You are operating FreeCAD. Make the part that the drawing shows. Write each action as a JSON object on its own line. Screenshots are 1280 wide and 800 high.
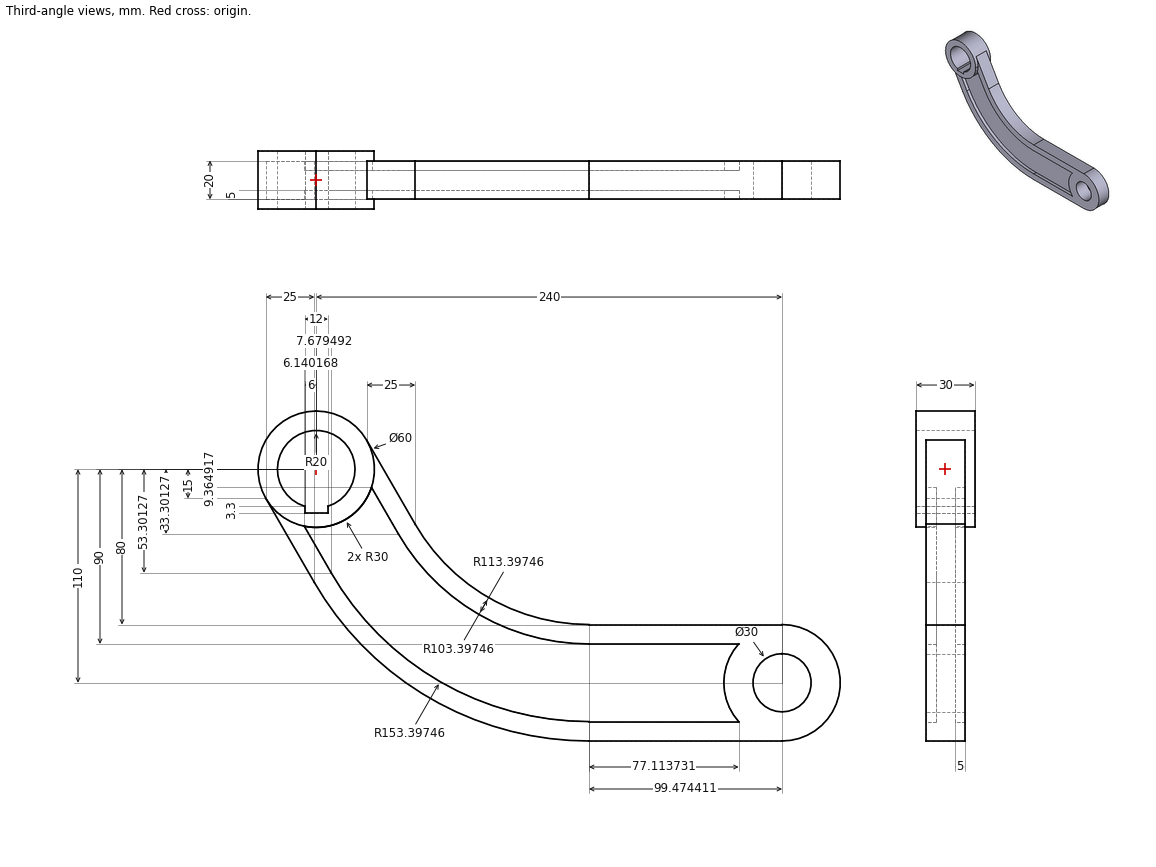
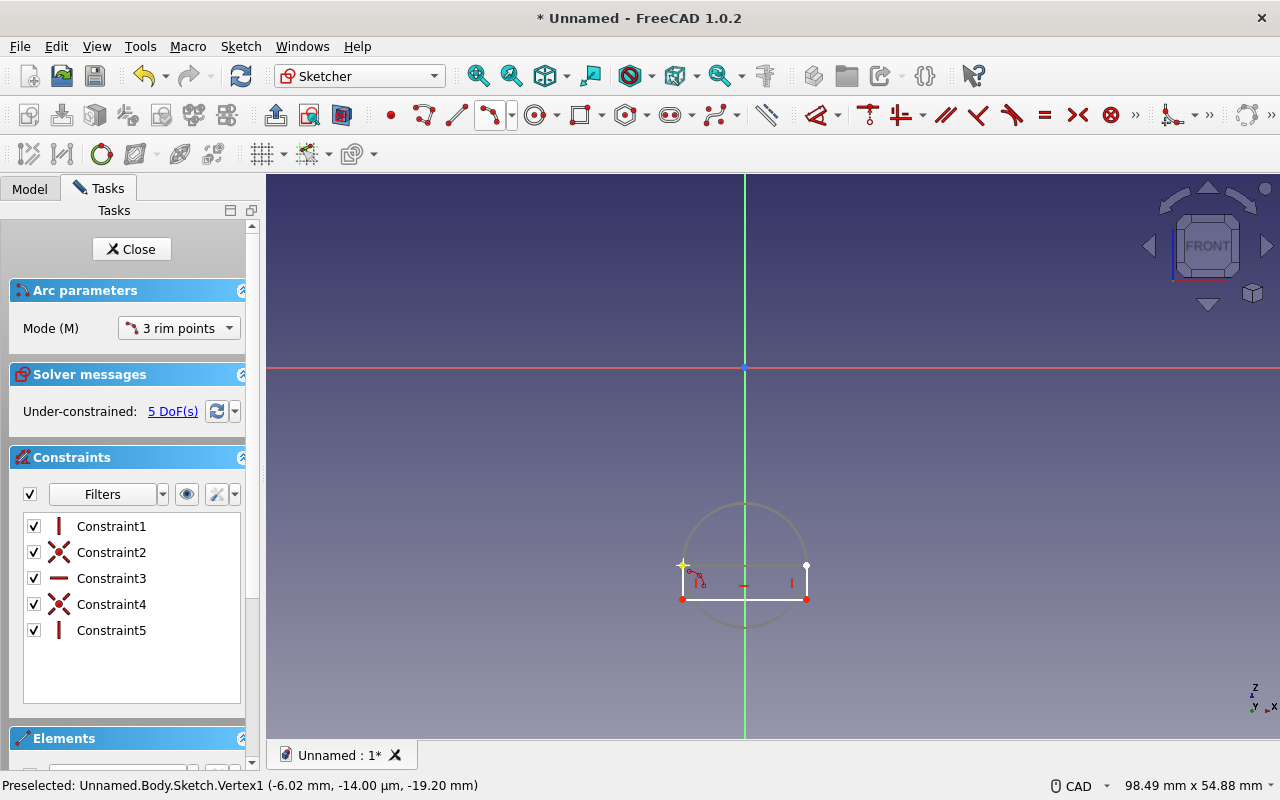
{"action": "scroll", "coordinate": [656, 565], "scroll_direction": "down", "scroll_amount": 3}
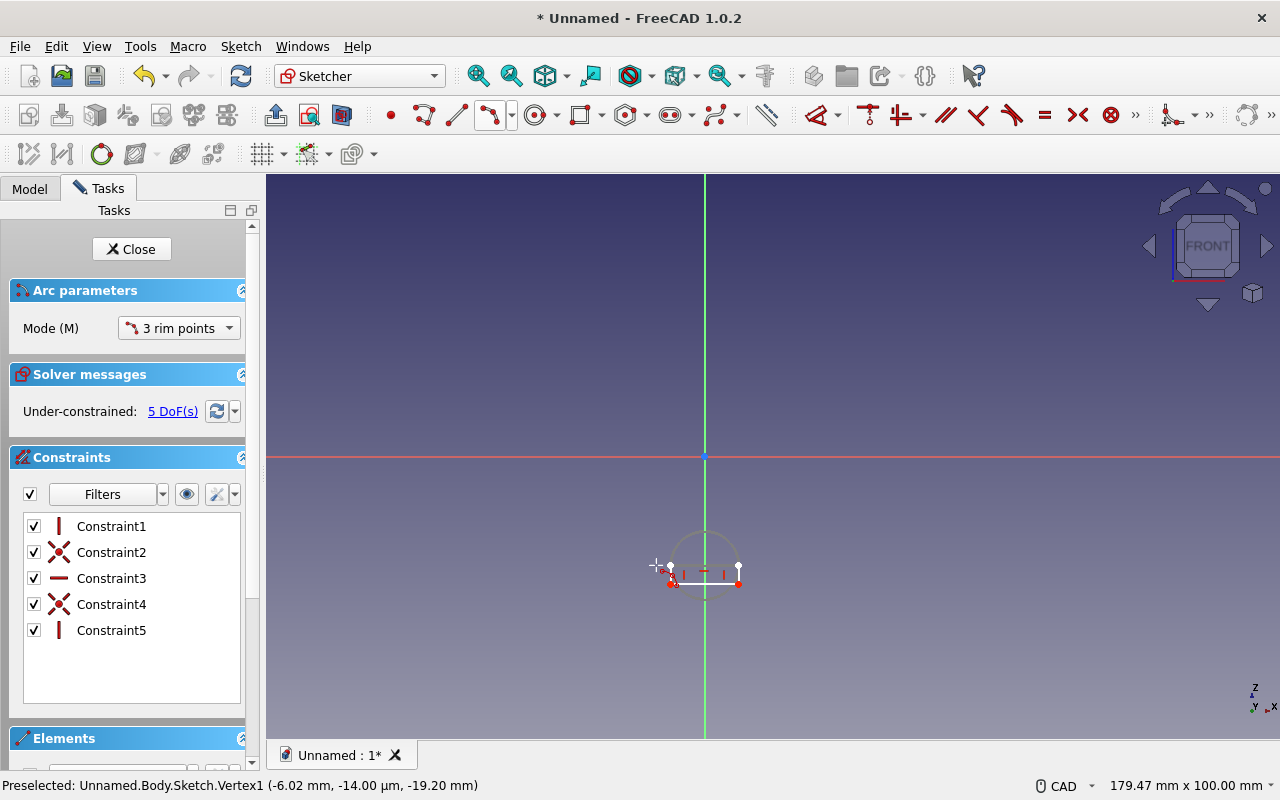
{"action": "left_click", "coordinate": [766, 362]}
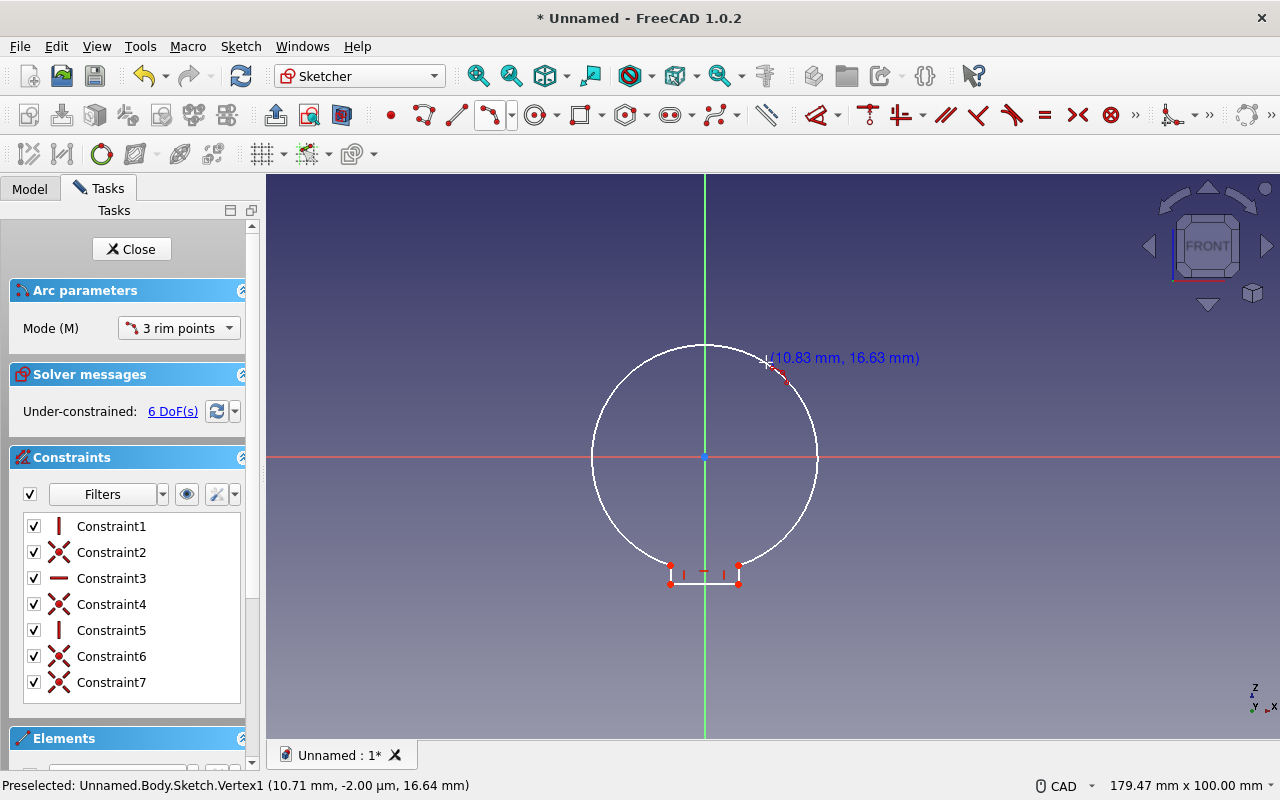
{"action": "left_click", "coordinate": [534, 116]}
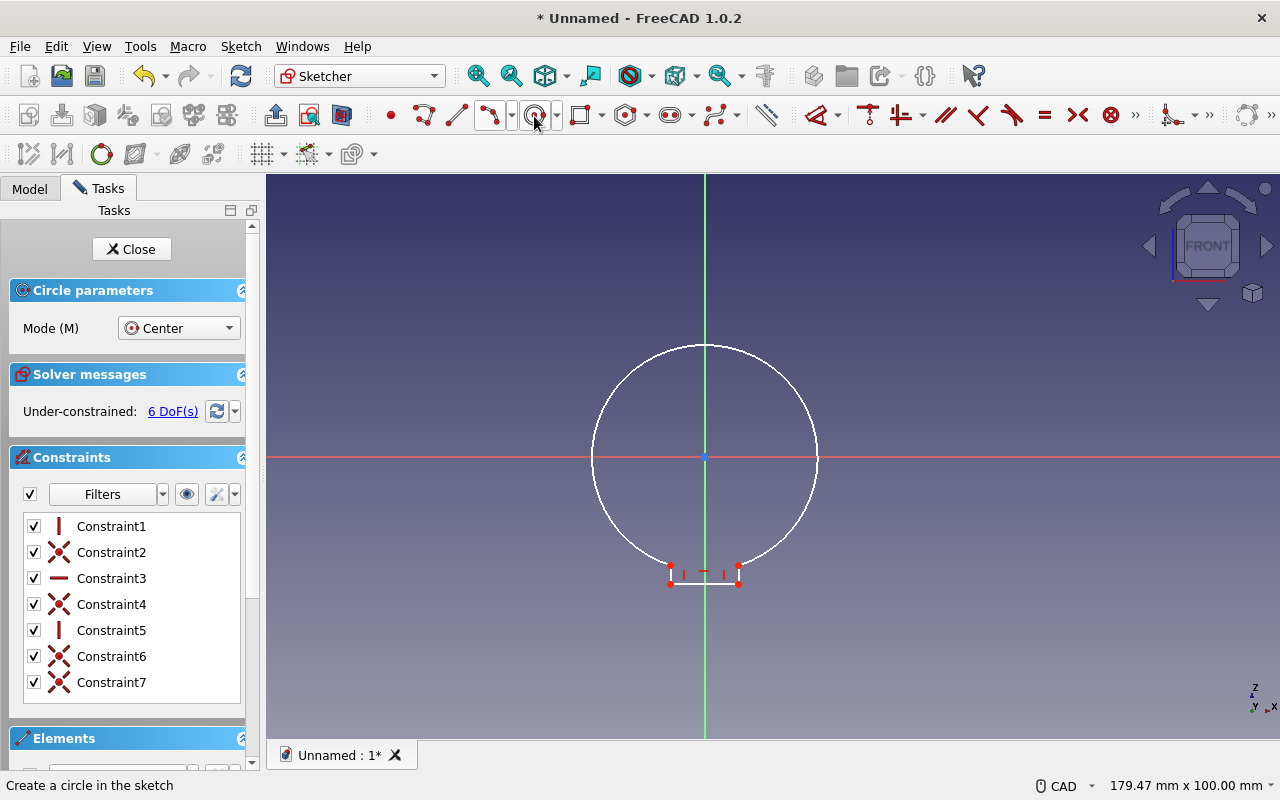
{"action": "left_click", "coordinate": [705, 457]}
{"action": "mouse_move", "coordinate": [825, 337]}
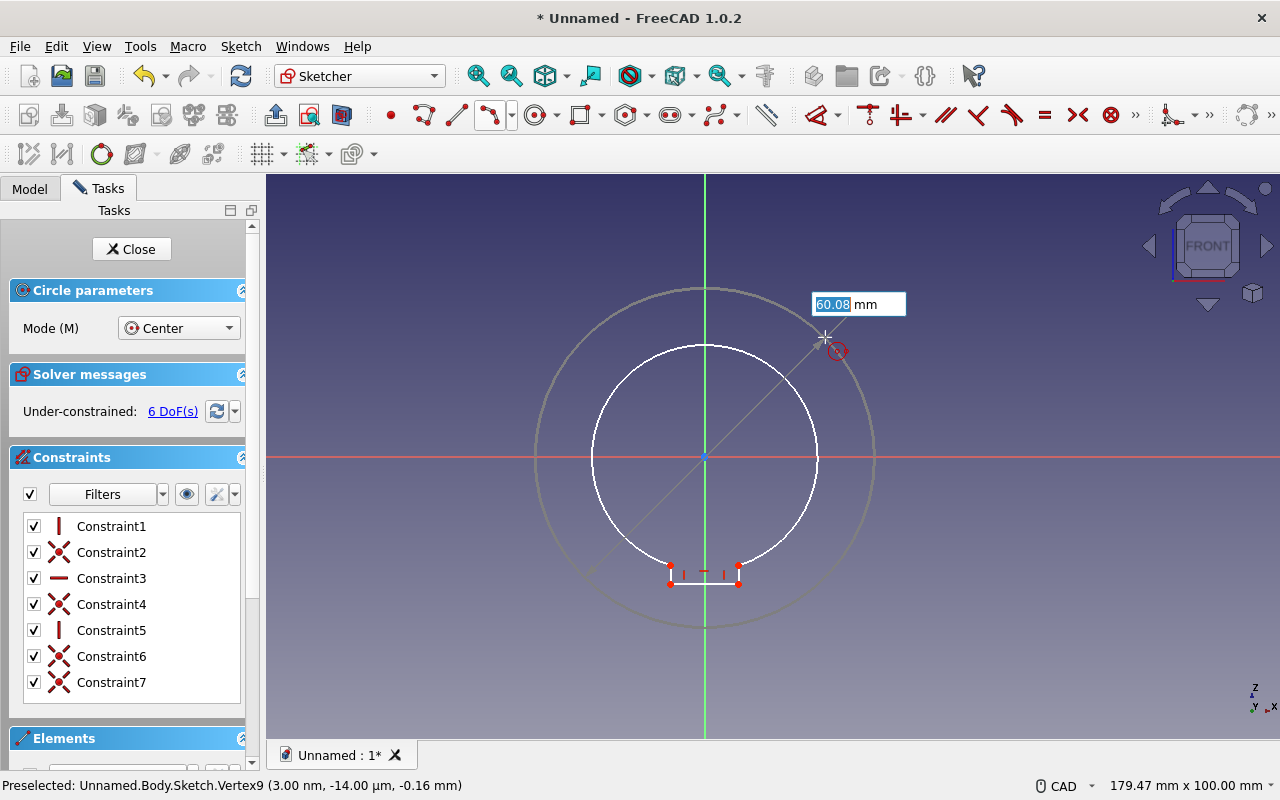
{"action": "type", "text": "60"}
{"action": "key", "text": "Return"}
{"action": "key", "text": "Escape"}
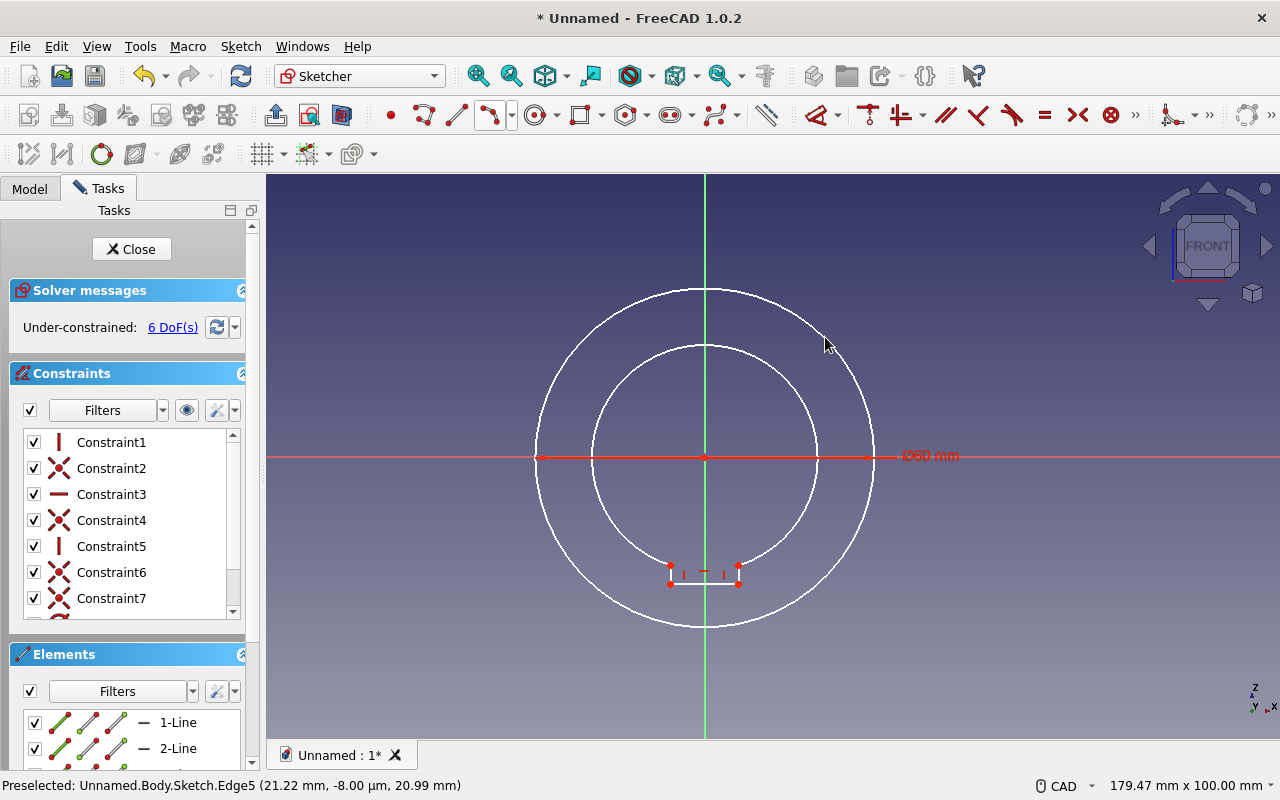
{"action": "left_click_drag", "start_coordinate": [695, 447], "coordinate": [715, 468]}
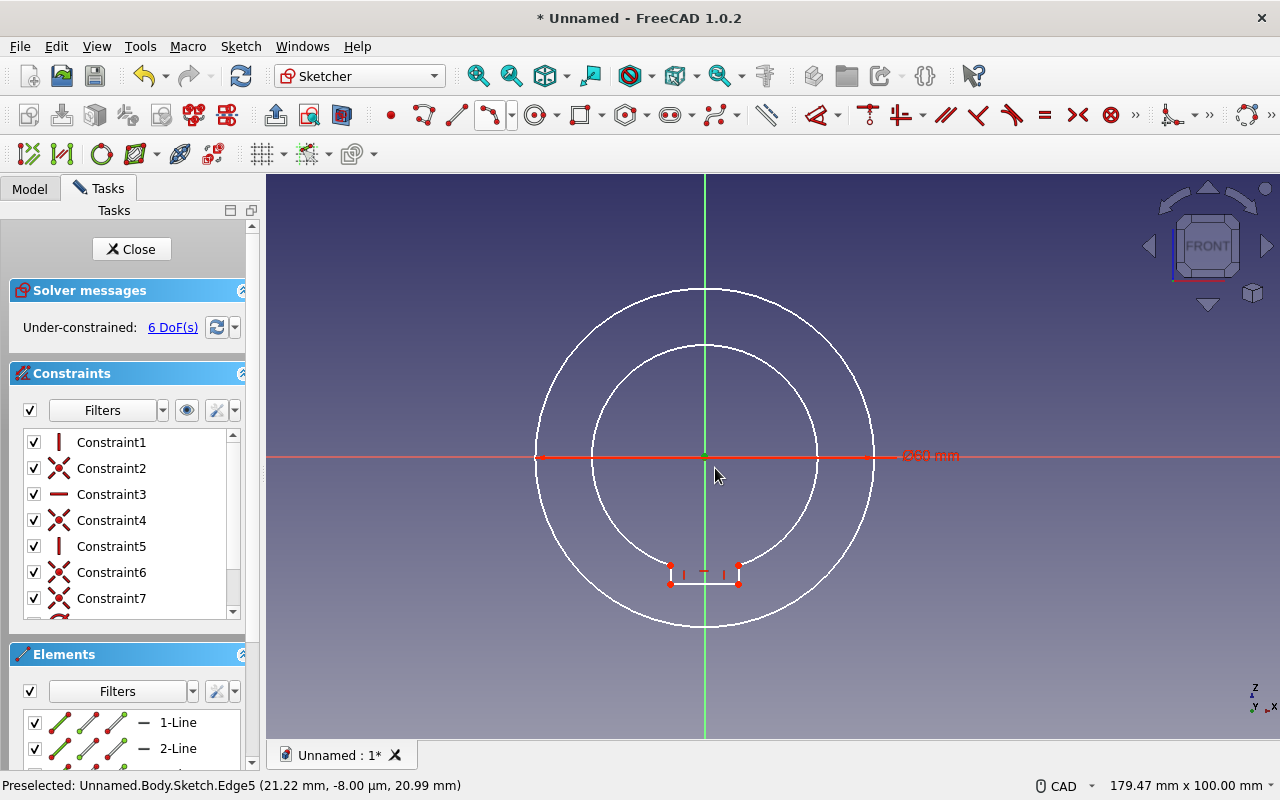
{"action": "left_click", "coordinate": [868, 116]}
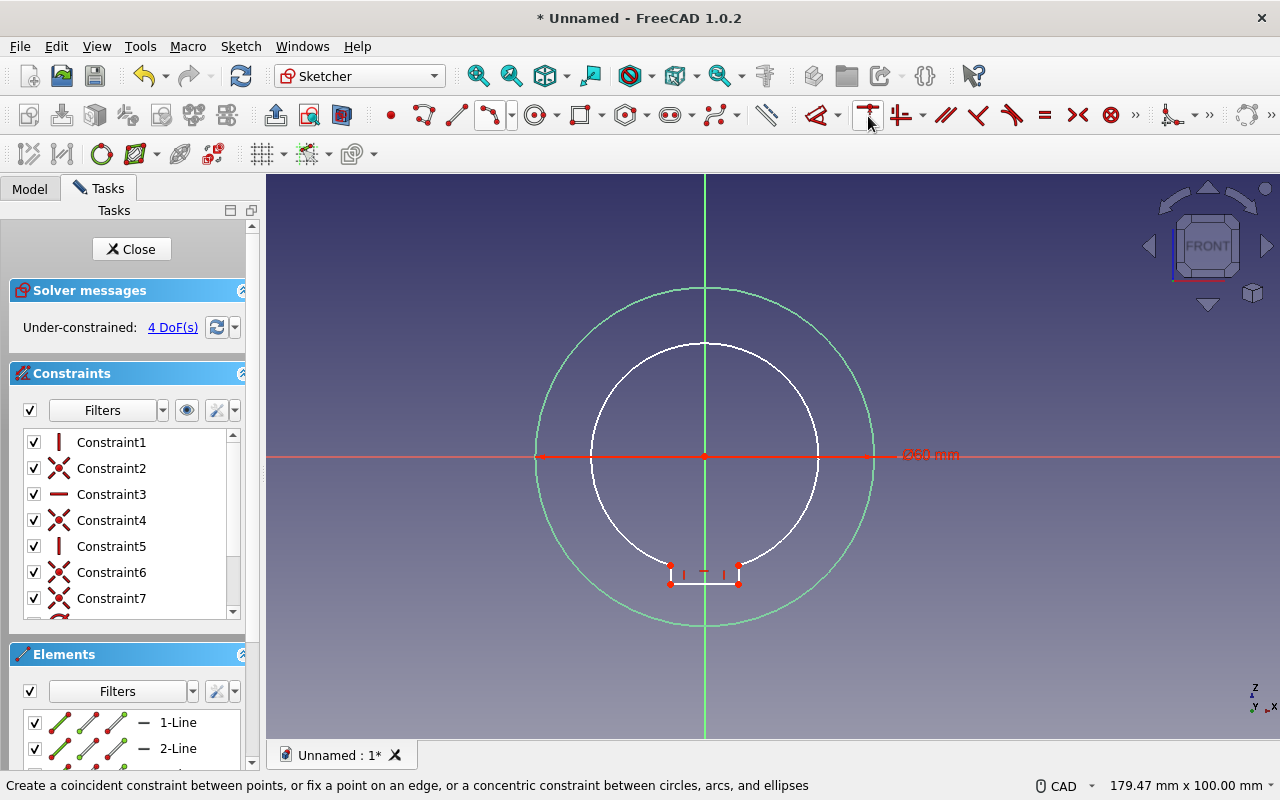
{"action": "left_click", "coordinate": [816, 116]}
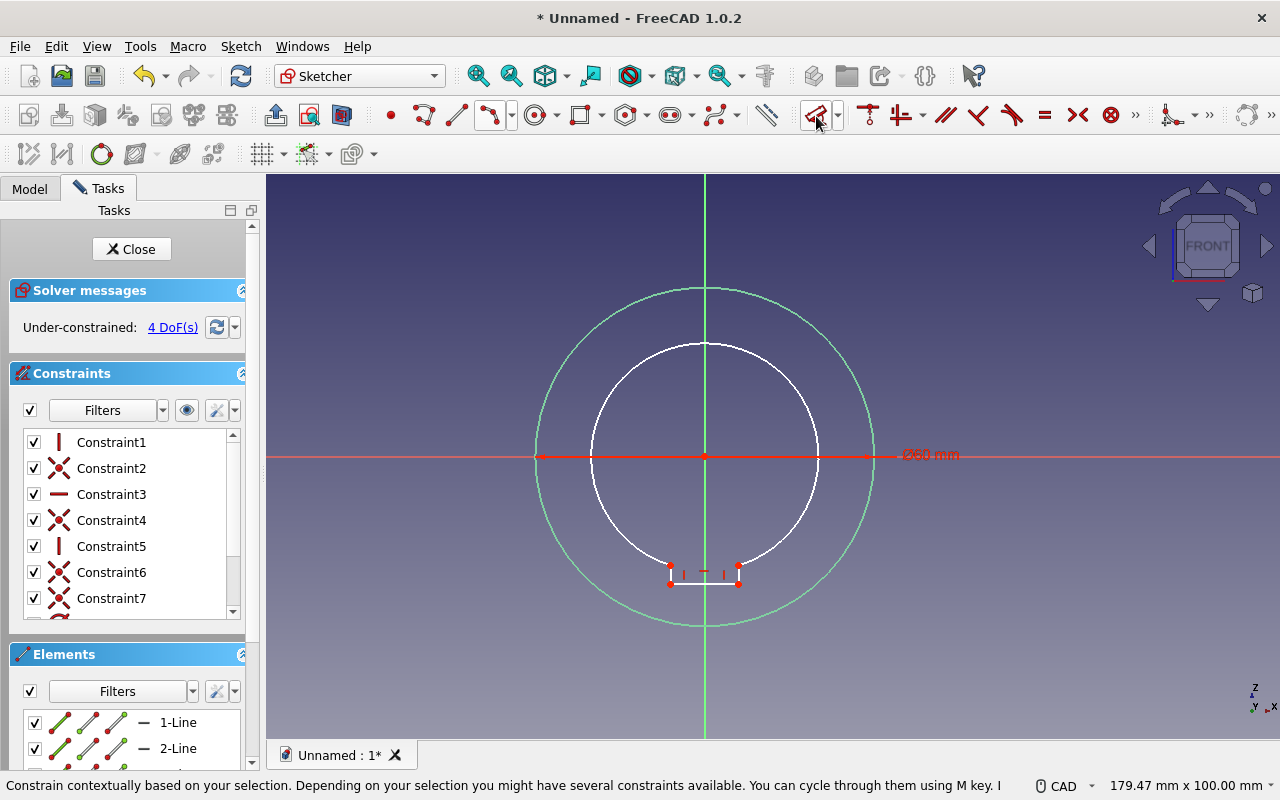
{"action": "left_click", "coordinate": [808, 409]}
{"action": "left_click", "coordinate": [837, 396]}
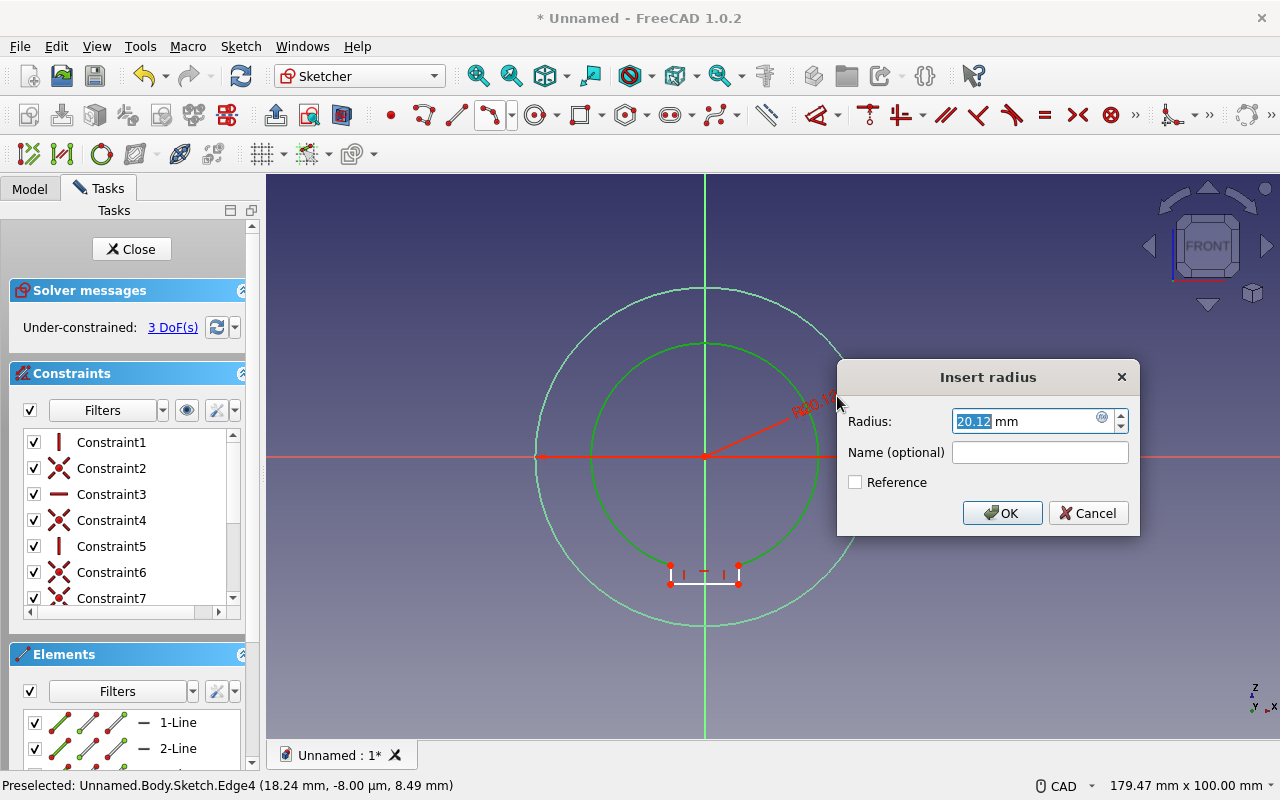
{"action": "type", "text": "20"}
{"action": "key", "text": "Return"}